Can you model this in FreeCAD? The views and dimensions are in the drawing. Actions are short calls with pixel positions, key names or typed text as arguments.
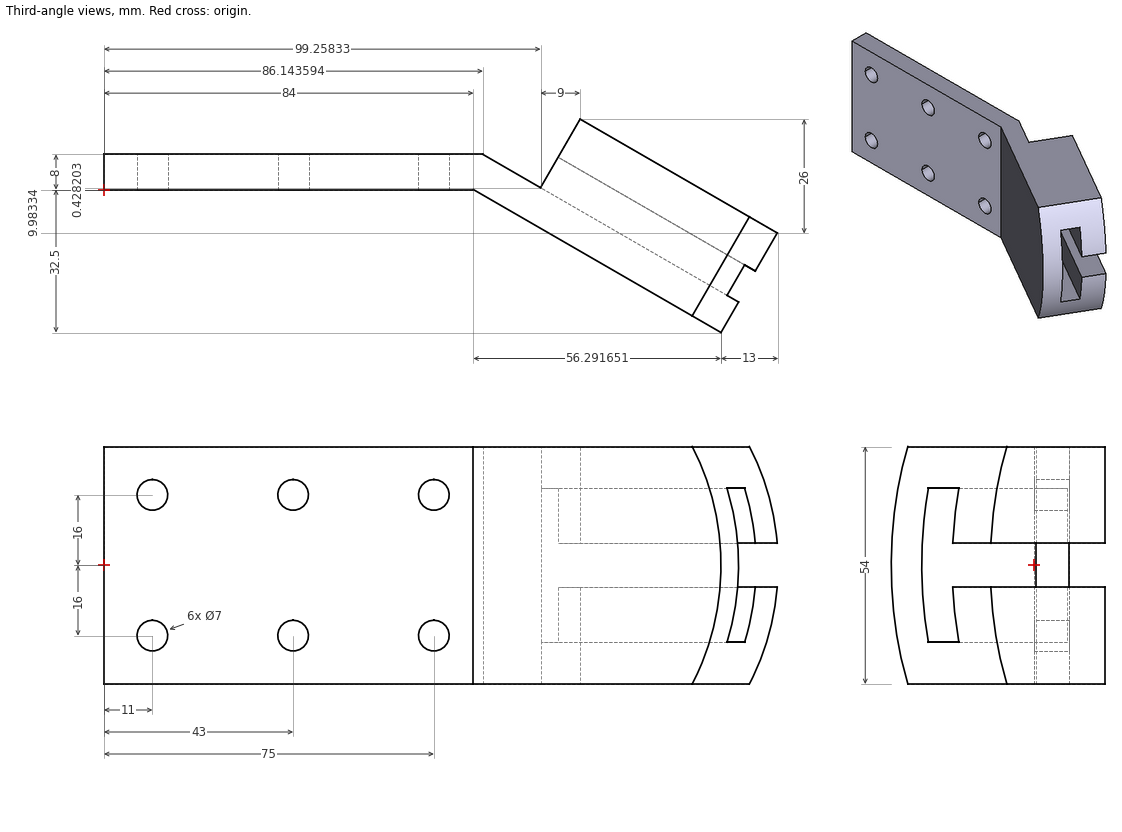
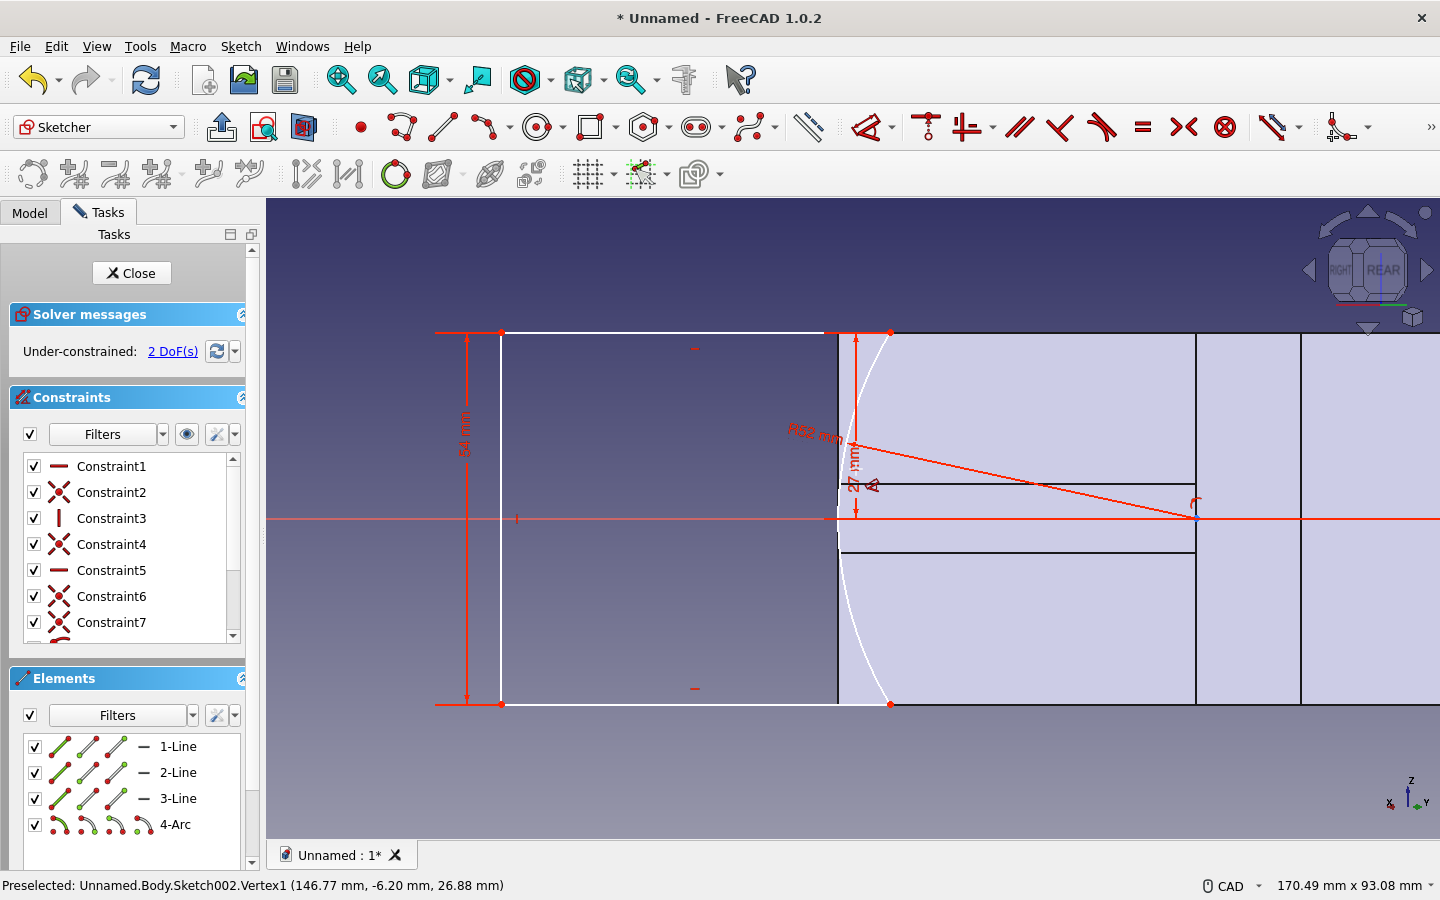
click(774, 333)
click(696, 299)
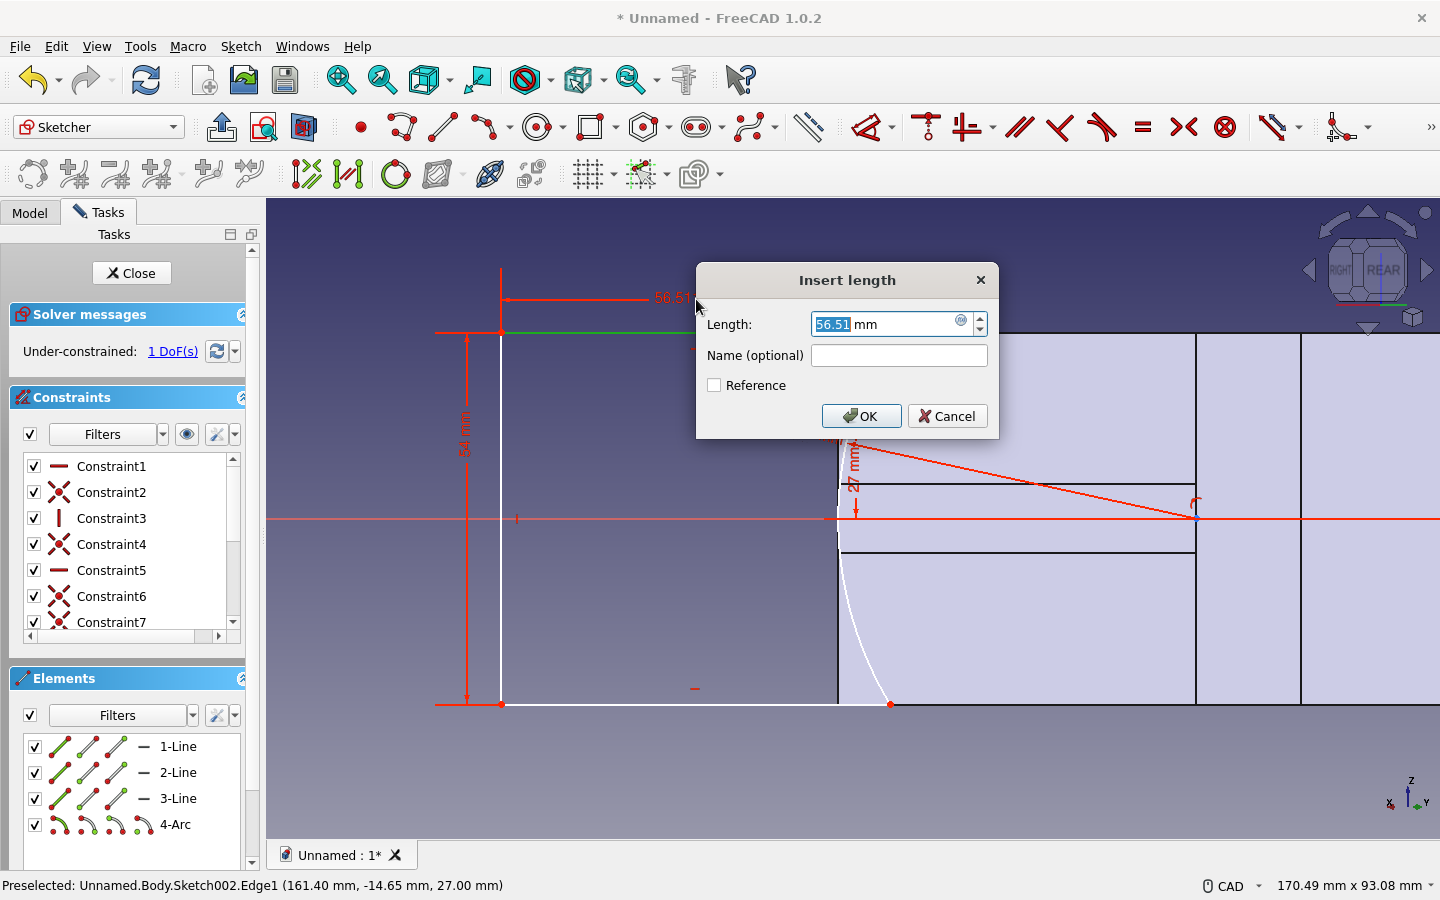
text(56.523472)
key(Return)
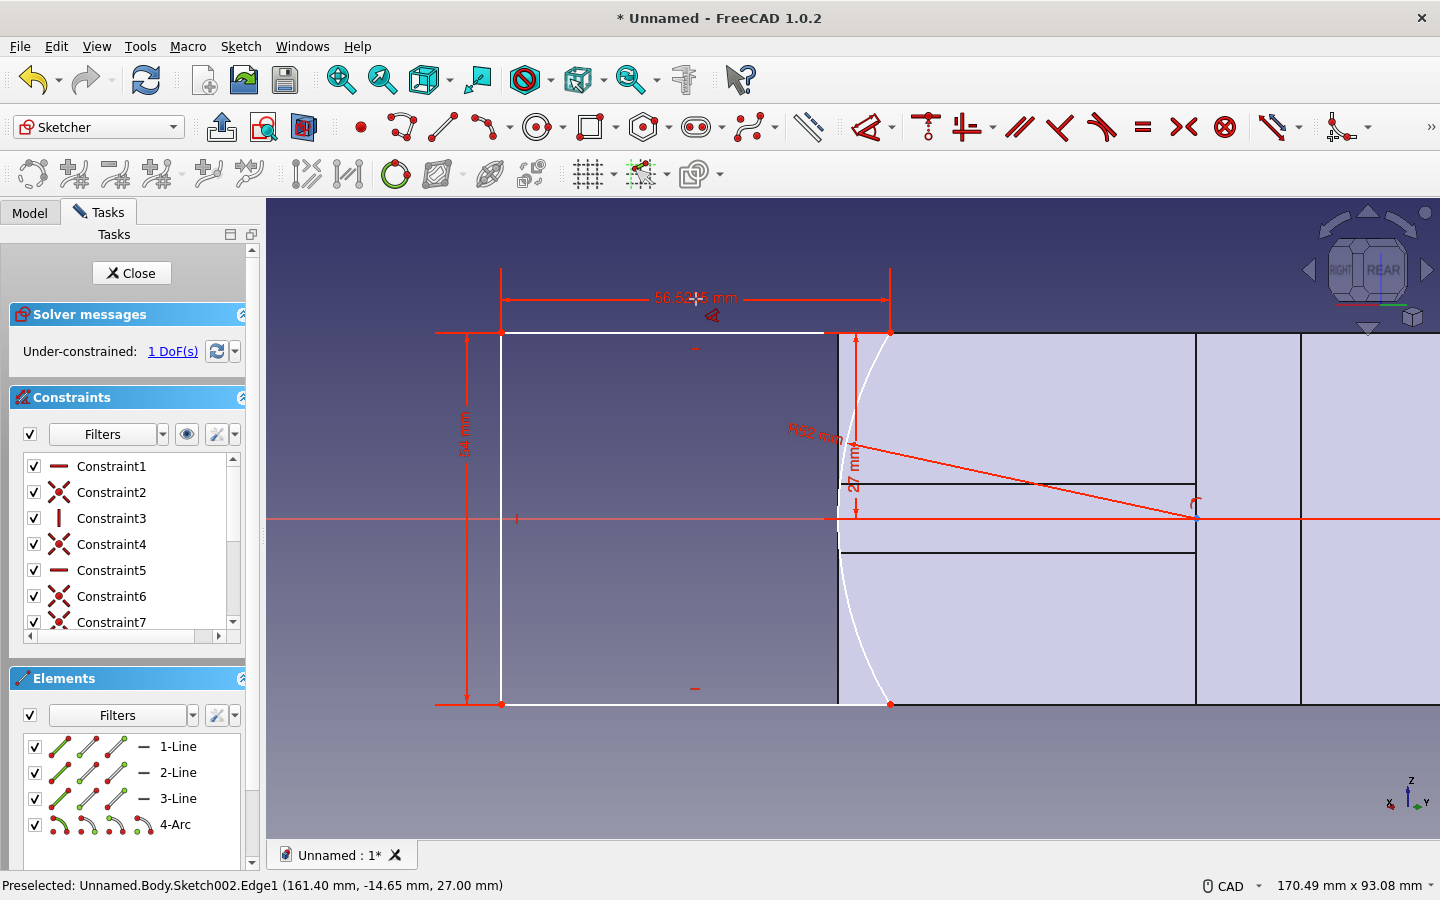
click(1196, 519)
click(1236, 485)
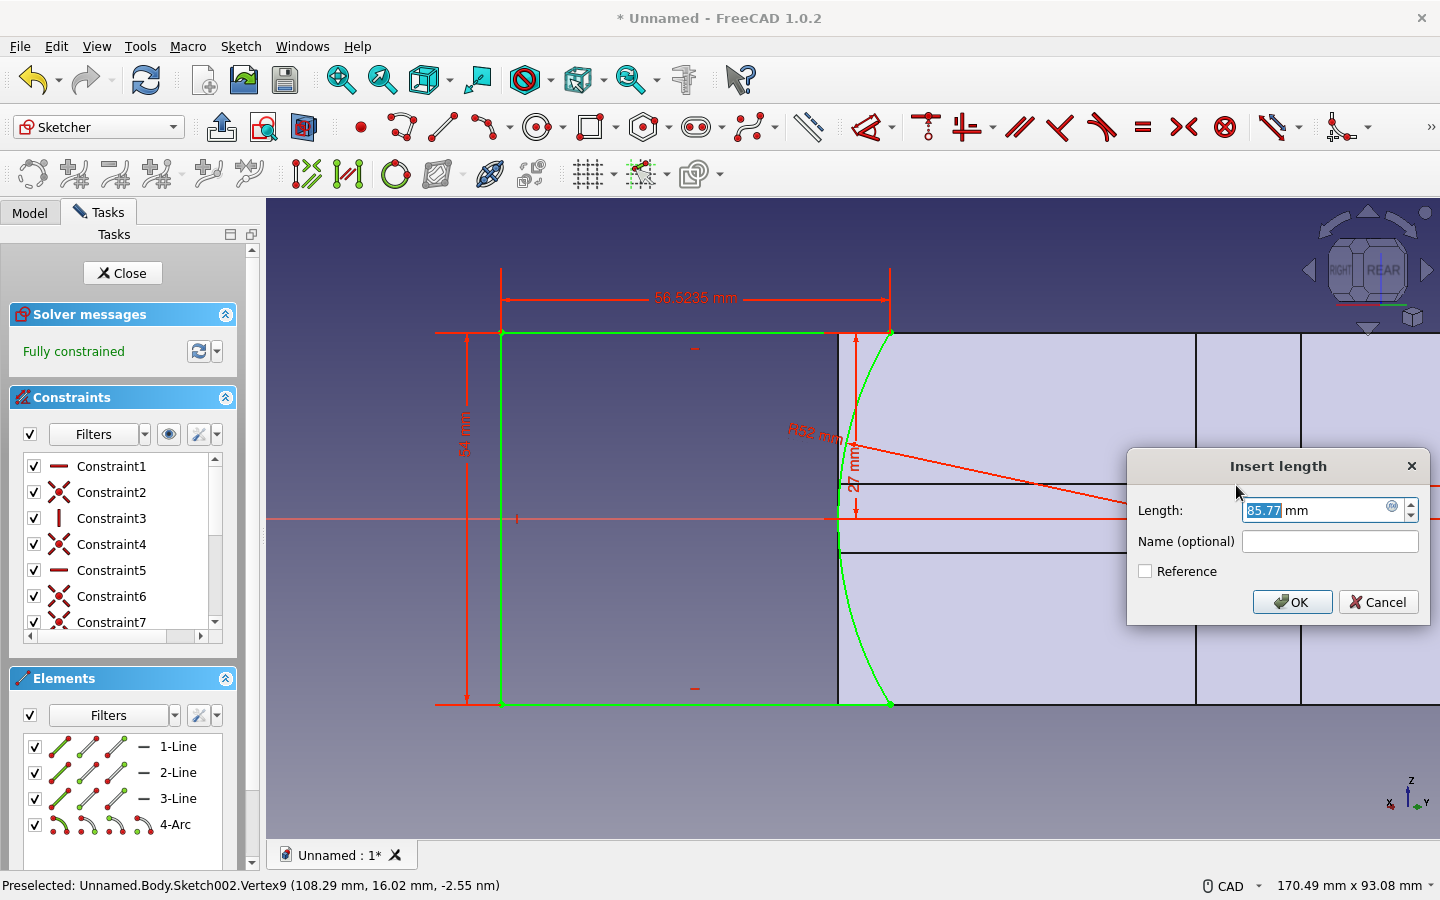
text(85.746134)
key(Return)
key(Escape)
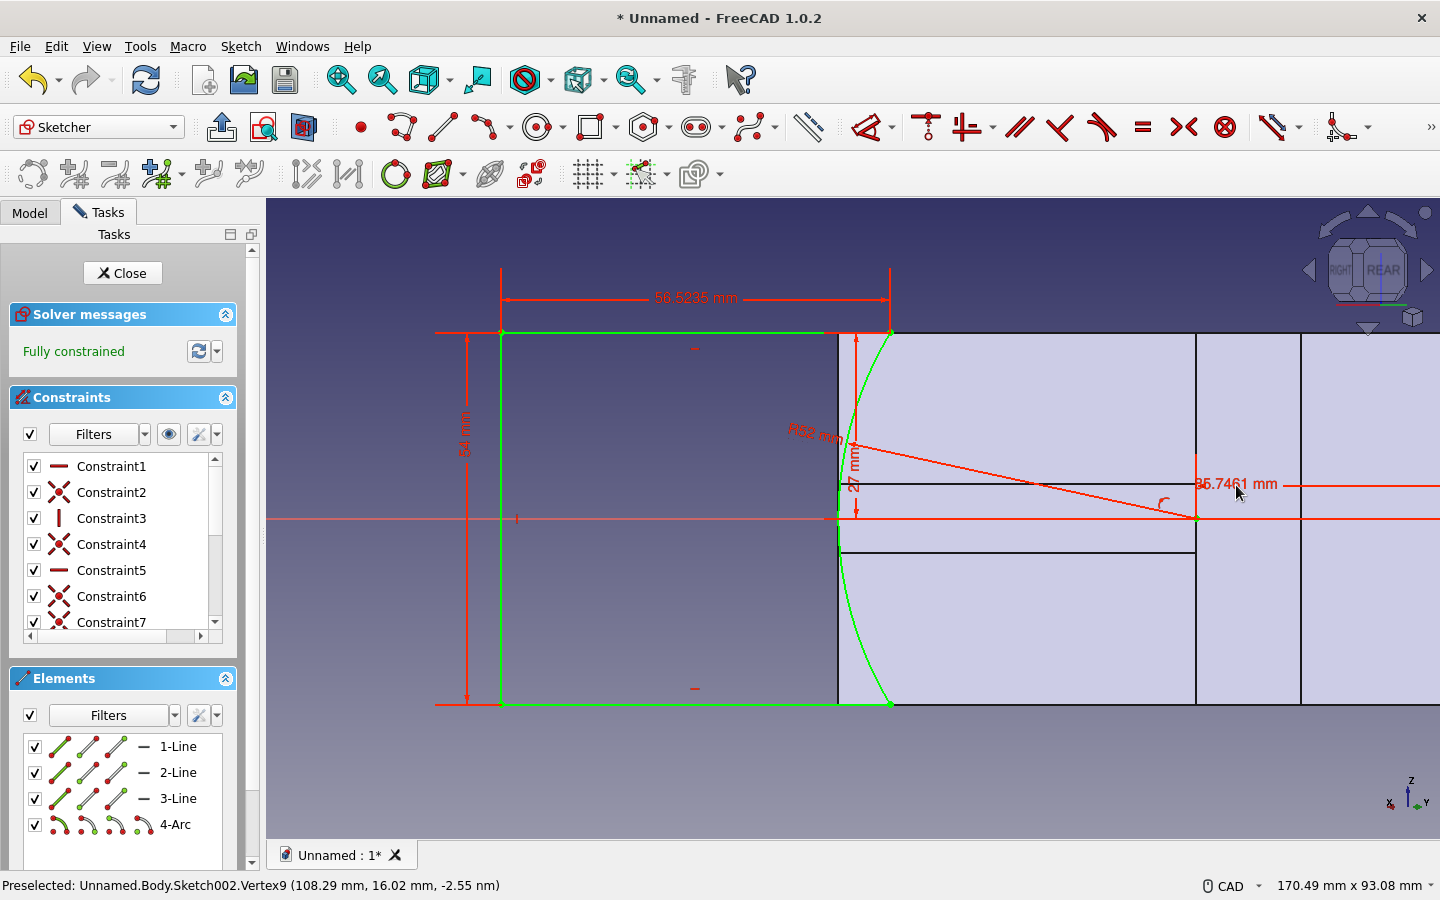
click(123, 273)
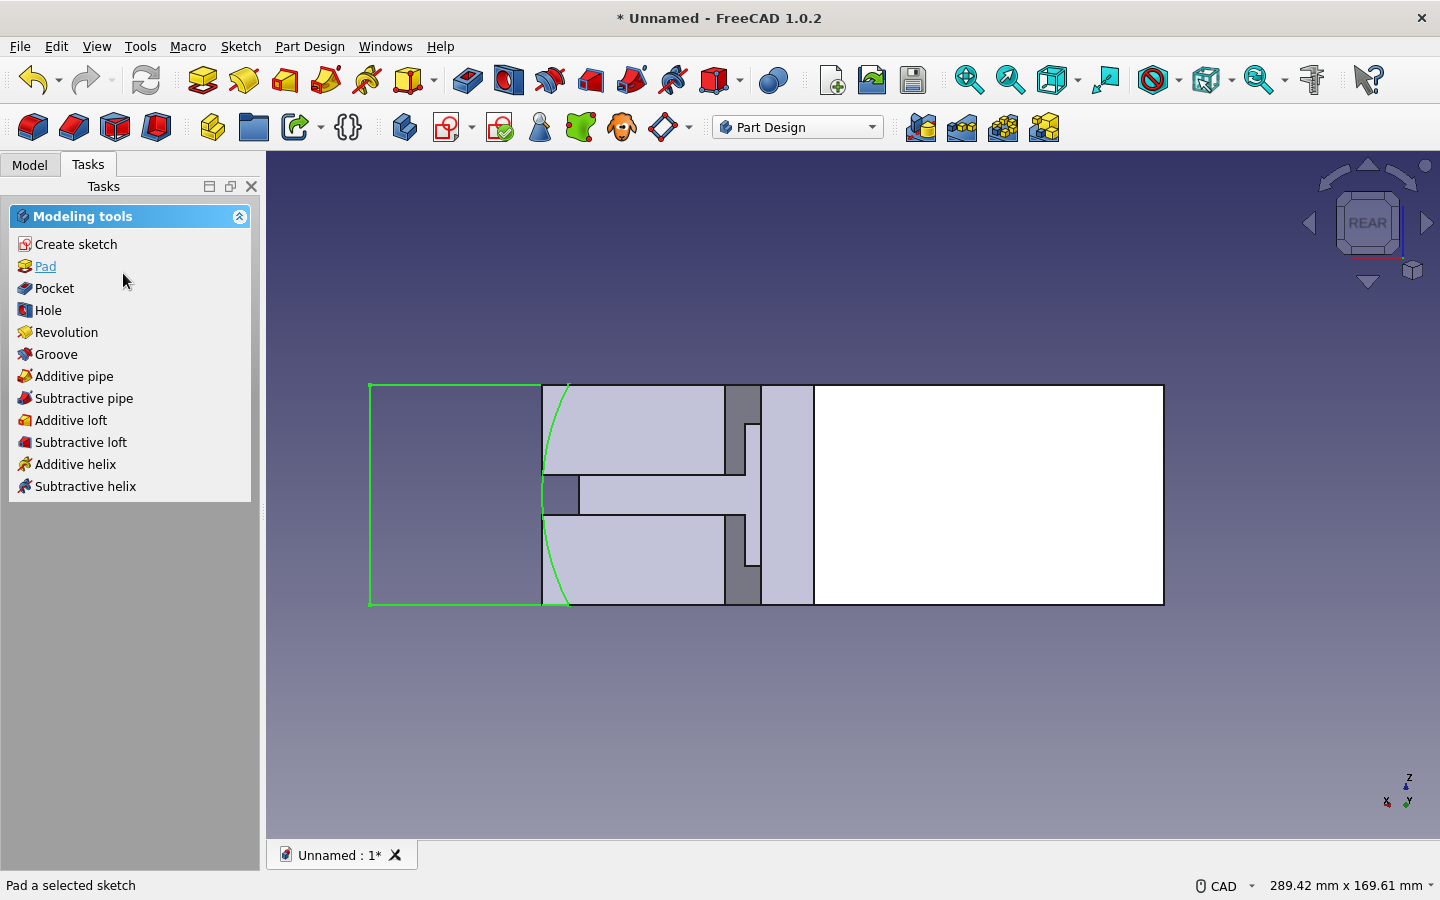
click(468, 80)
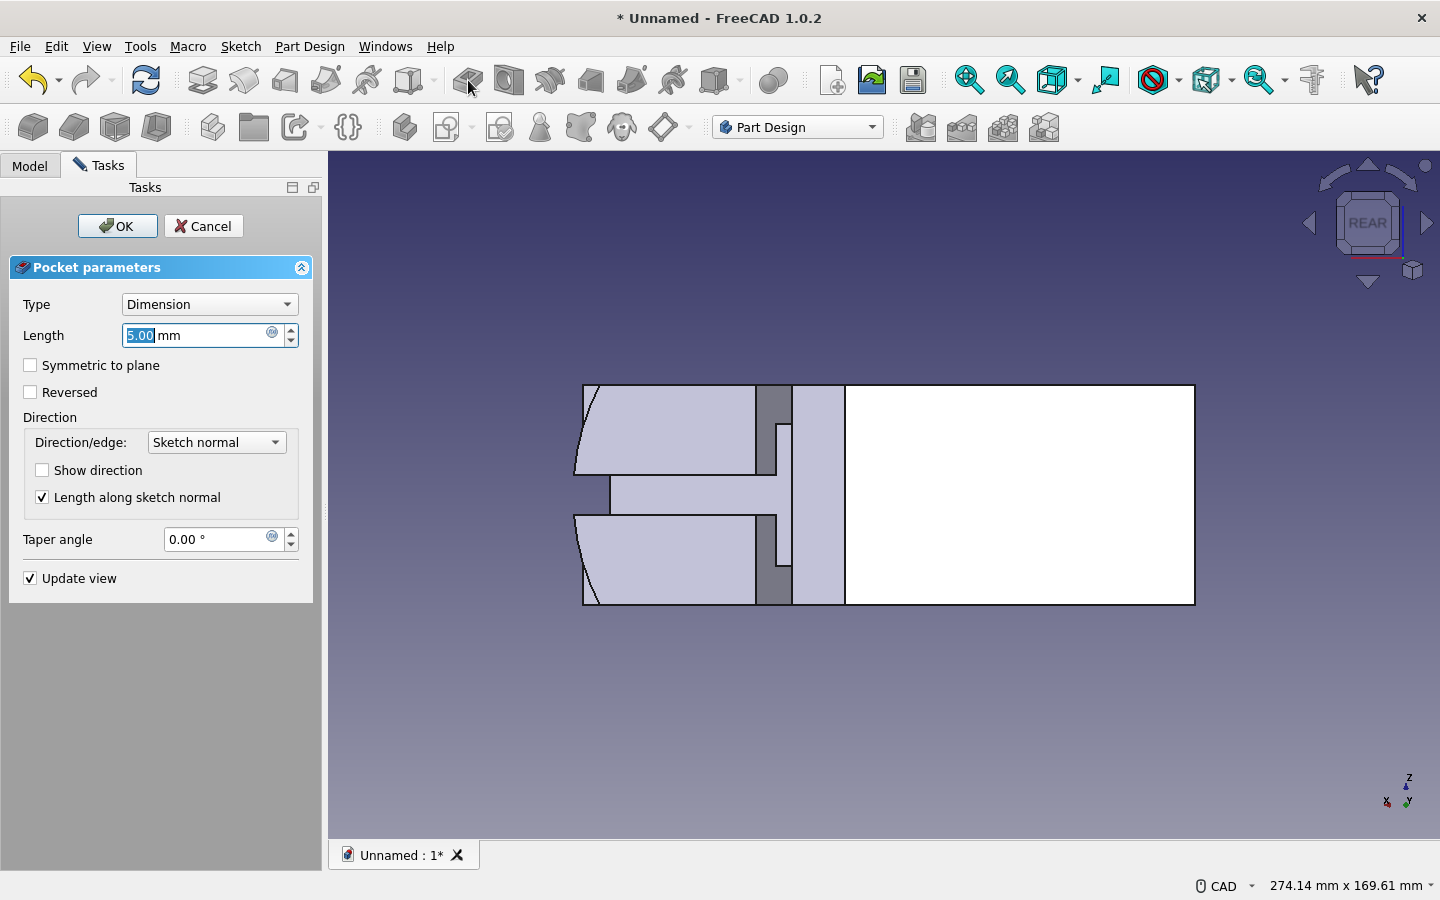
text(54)
key(Tab)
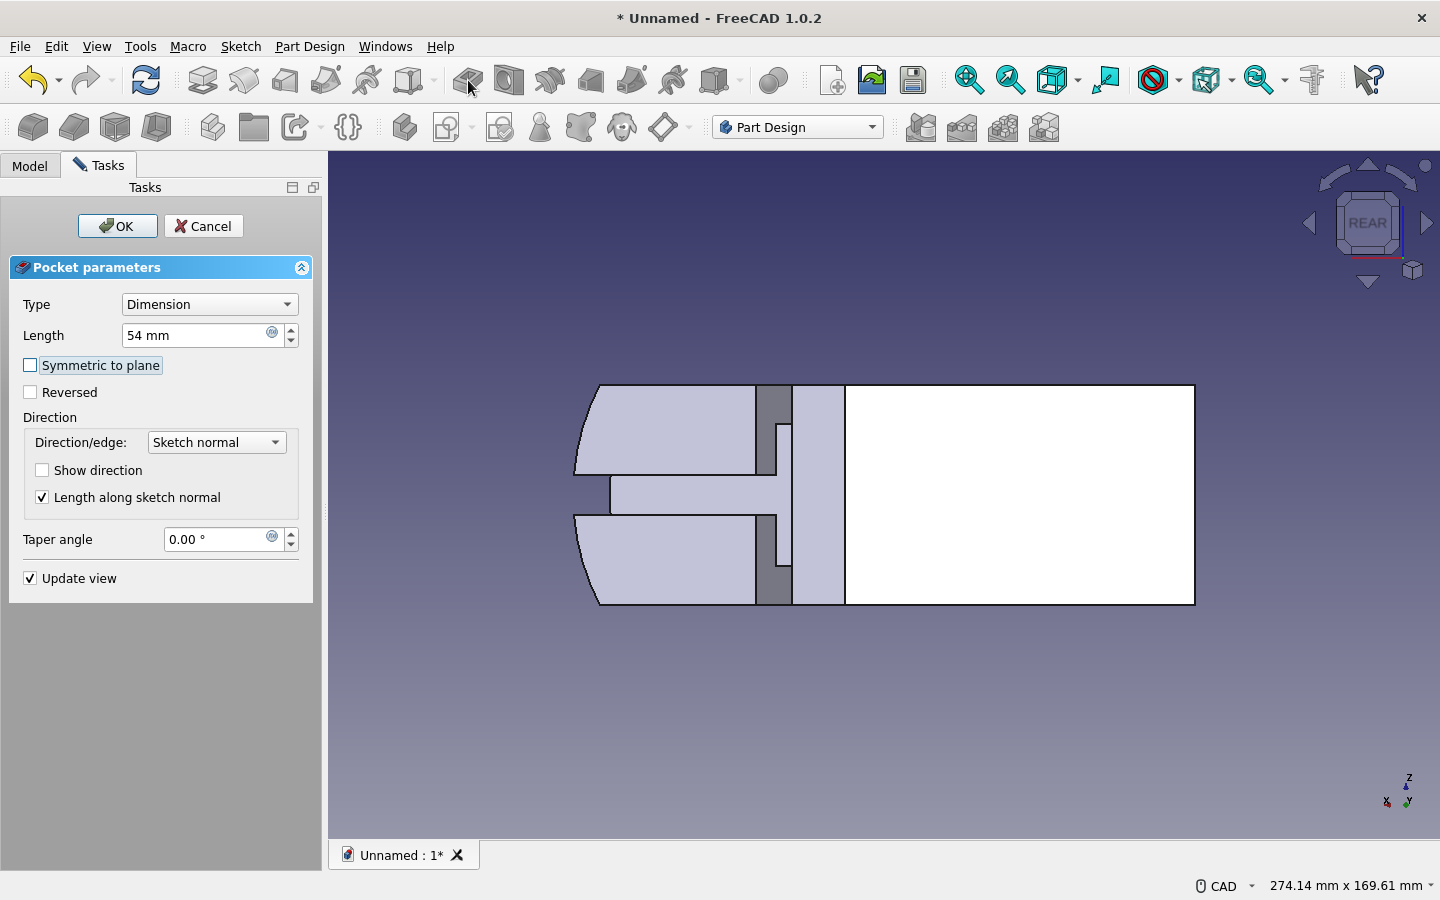
click(118, 226)